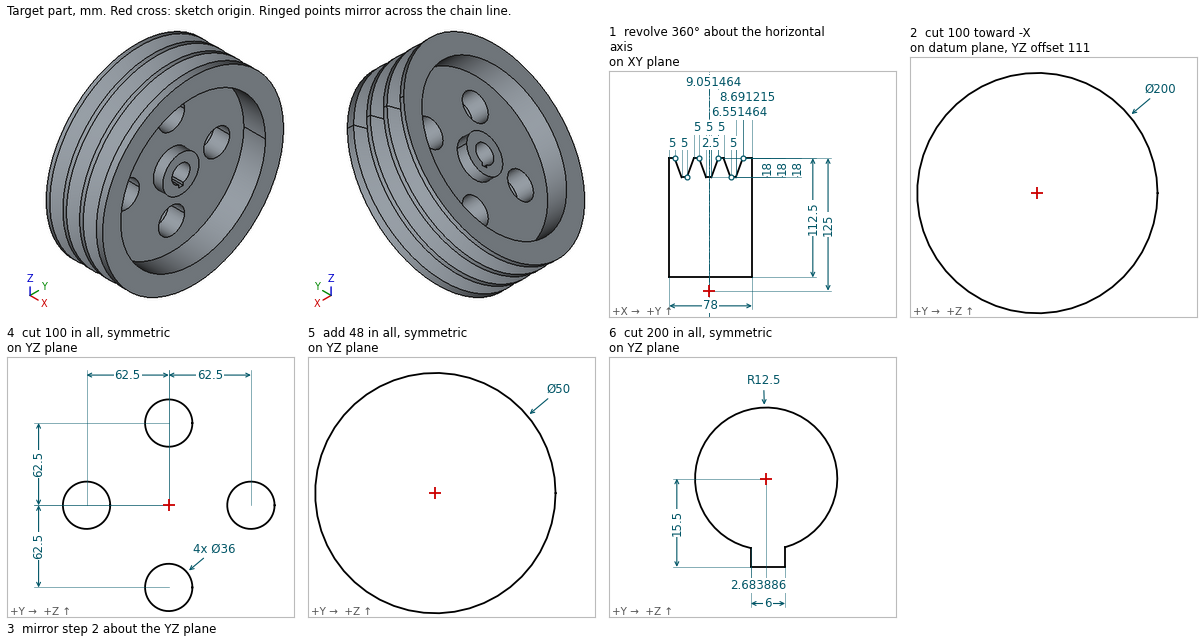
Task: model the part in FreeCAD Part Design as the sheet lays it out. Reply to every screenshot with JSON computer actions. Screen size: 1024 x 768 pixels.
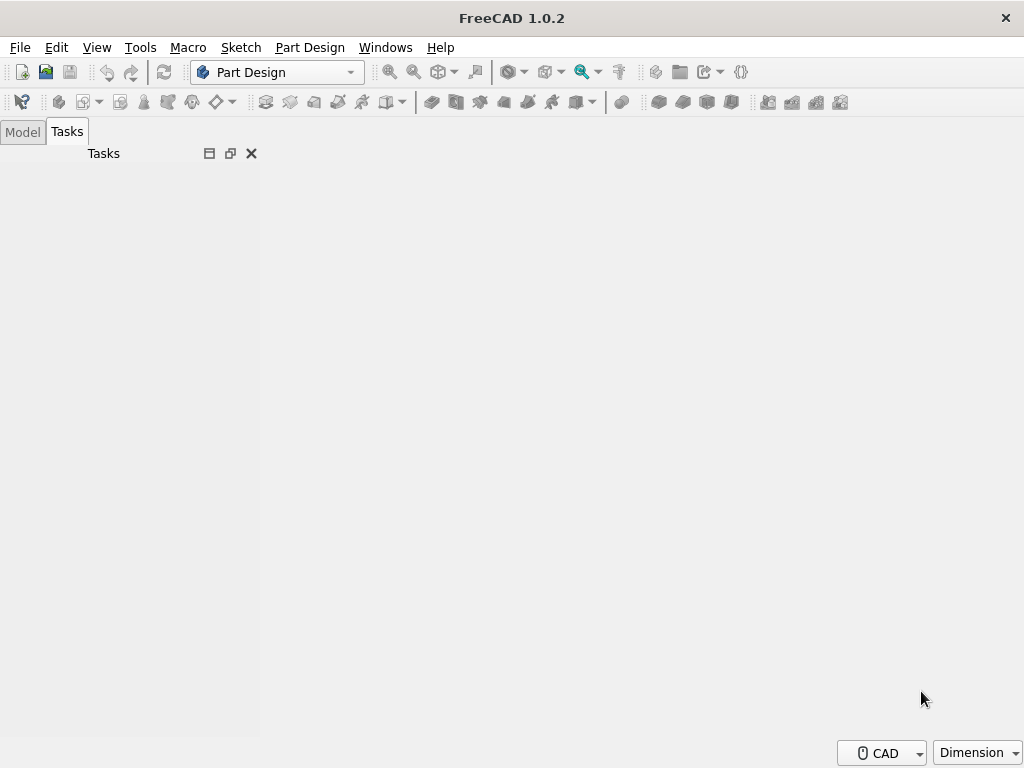
{"action": "left_click", "coordinate": [22, 72]}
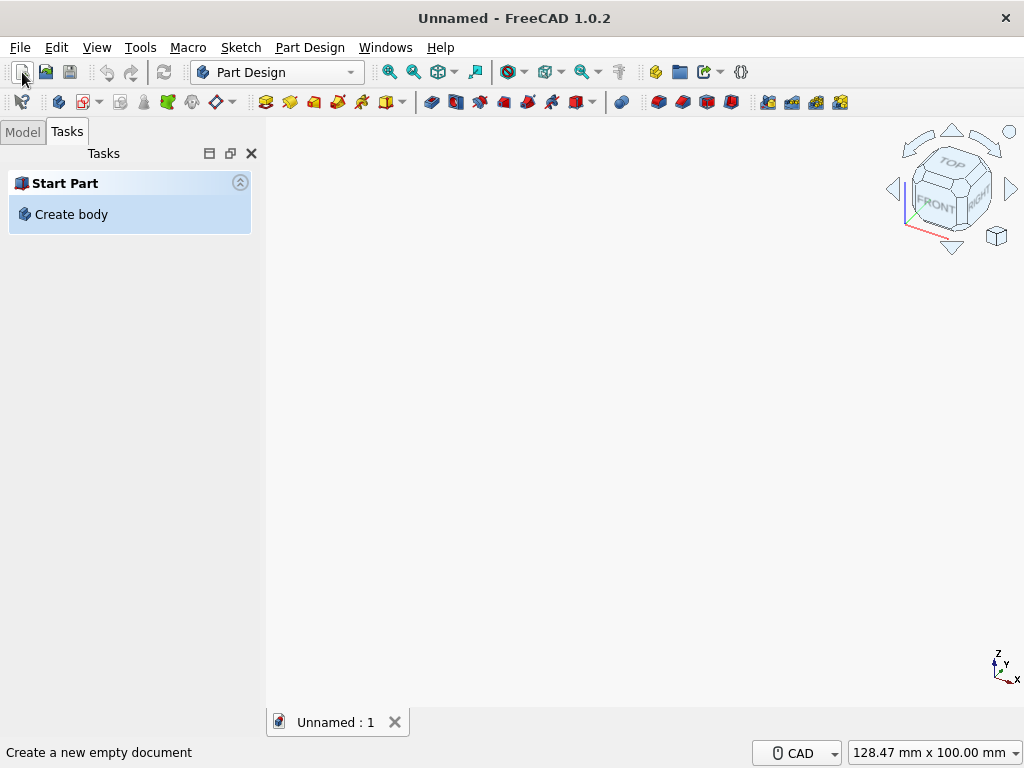
{"action": "left_click", "coordinate": [84, 102]}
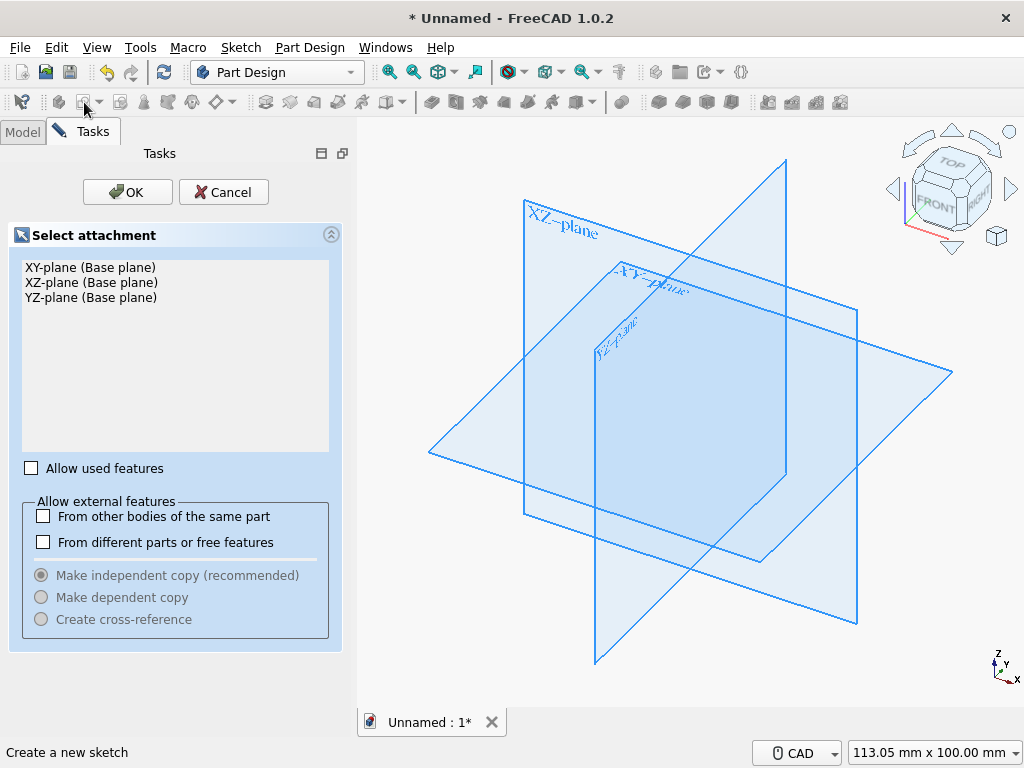
{"action": "left_click", "coordinate": [82, 268]}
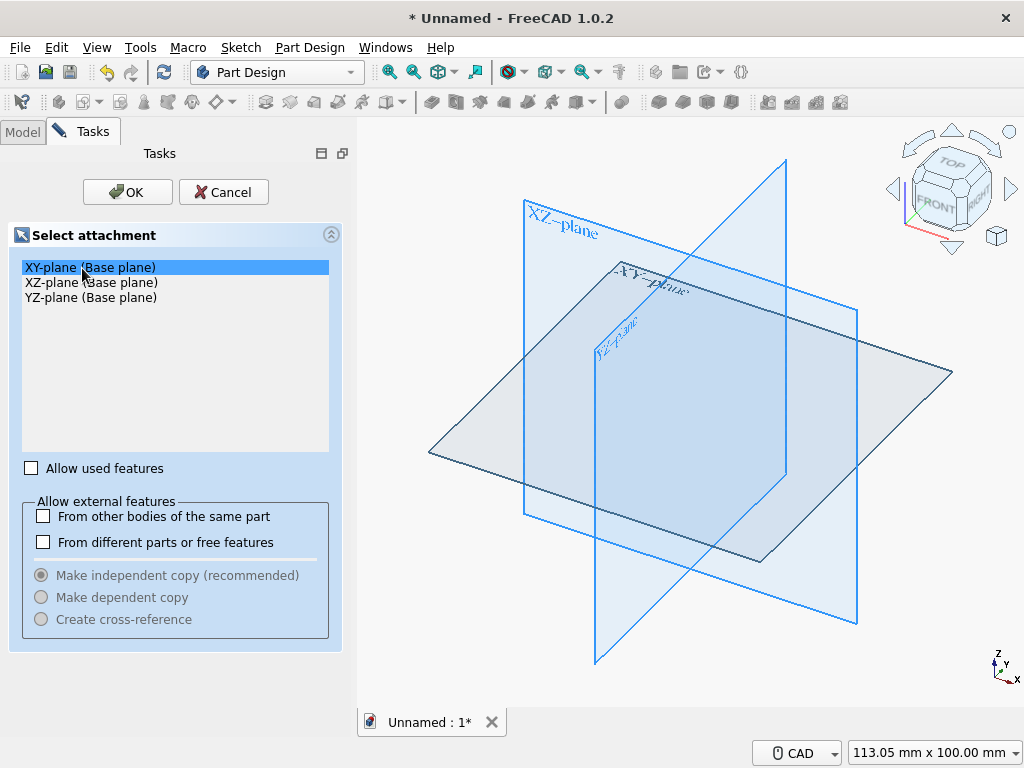
{"action": "left_click", "coordinate": [128, 192]}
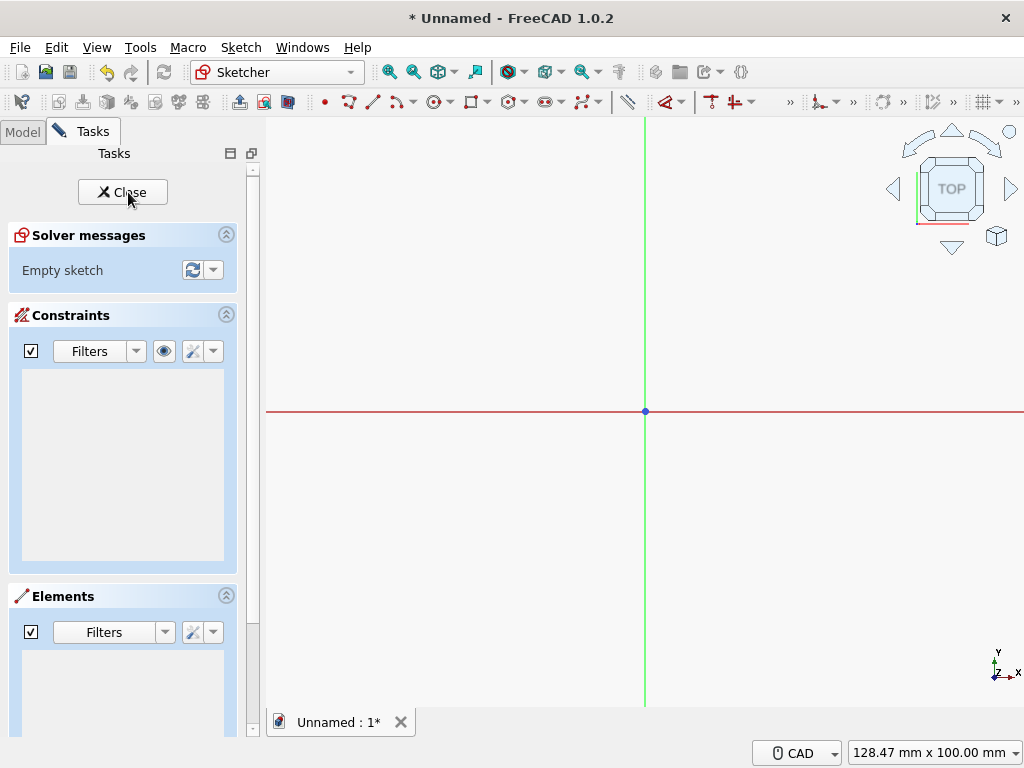
{"action": "scroll", "coordinate": [512, 679], "scroll_direction": "down", "scroll_amount": 4}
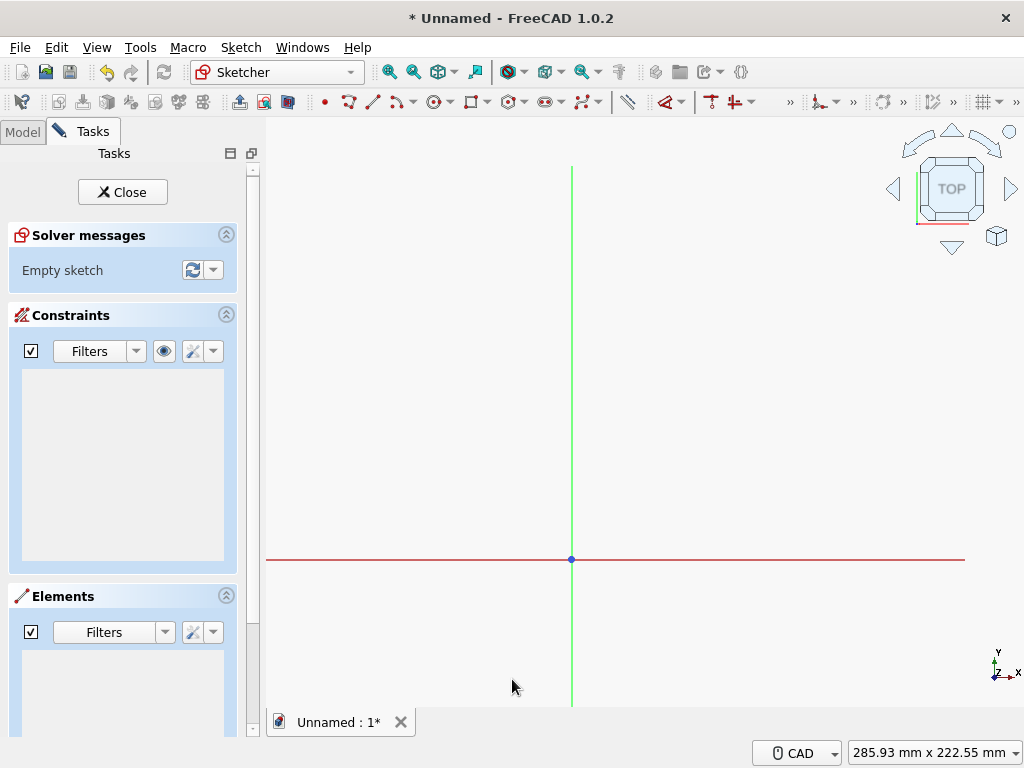
{"action": "left_click", "coordinate": [350, 102]}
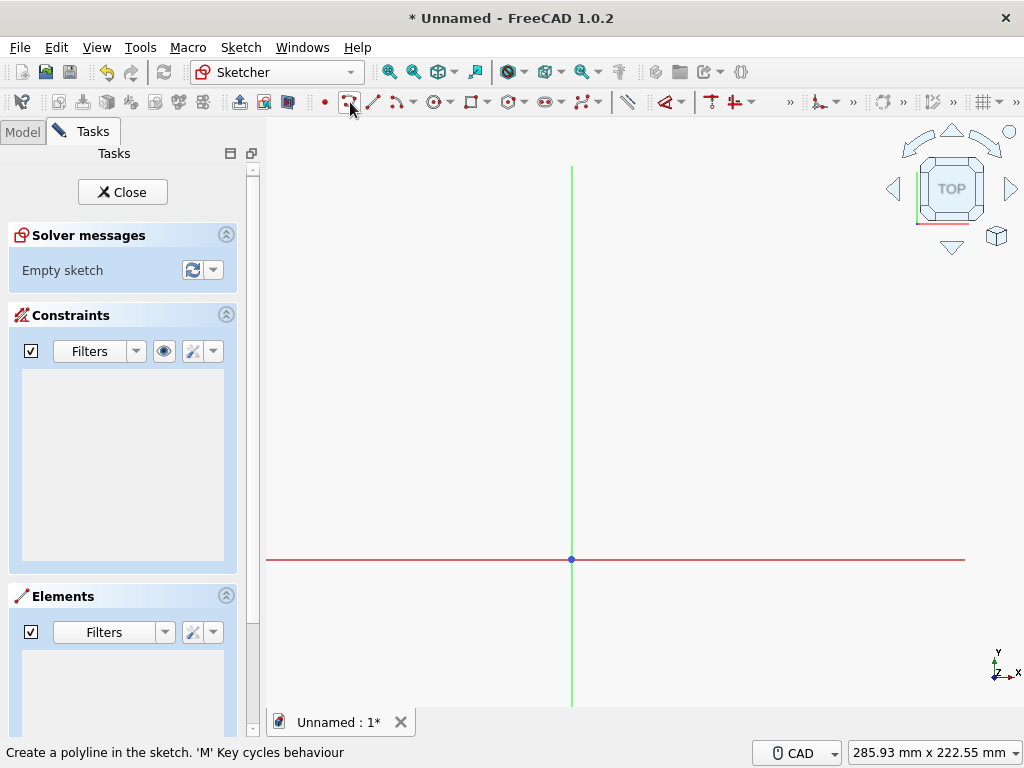
{"action": "left_click", "coordinate": [473, 526]}
{"action": "left_click", "coordinate": [680, 526]}
{"action": "left_click", "coordinate": [680, 228]}
{"action": "left_click", "coordinate": [657, 228]}
{"action": "left_click", "coordinate": [640, 276]}
{"action": "left_click", "coordinate": [627, 276]}
{"action": "left_click", "coordinate": [609, 228]}
{"action": "left_click", "coordinate": [596, 228]}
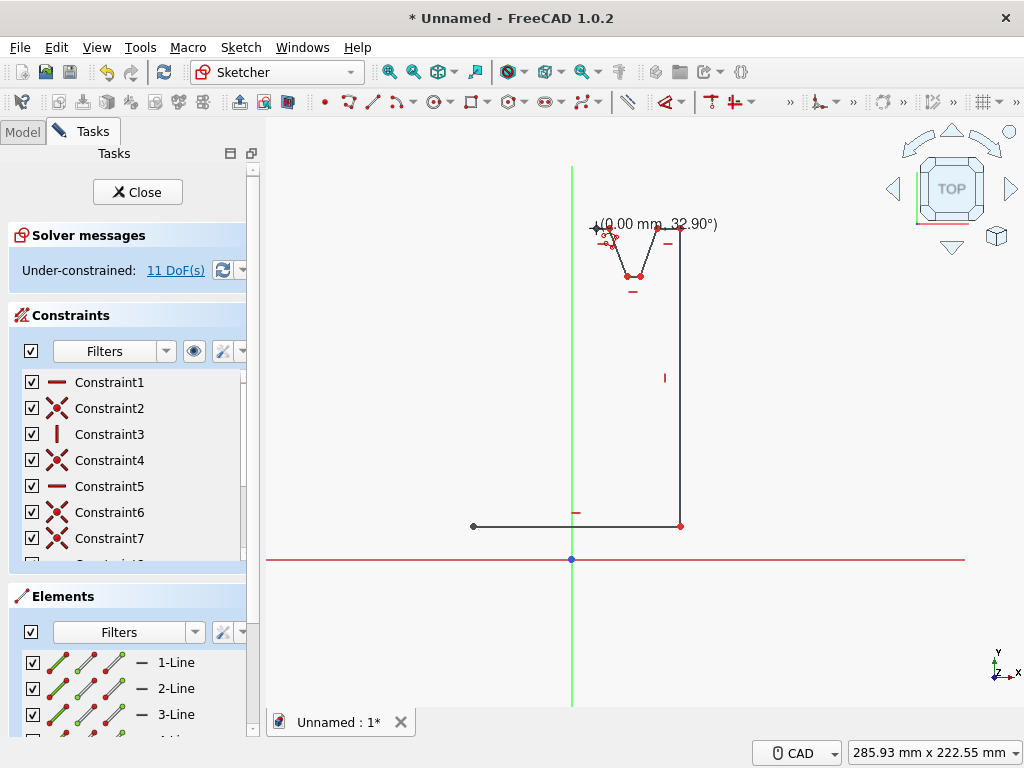
{"action": "scroll", "coordinate": [579, 276], "scroll_direction": "up", "scroll_amount": 5}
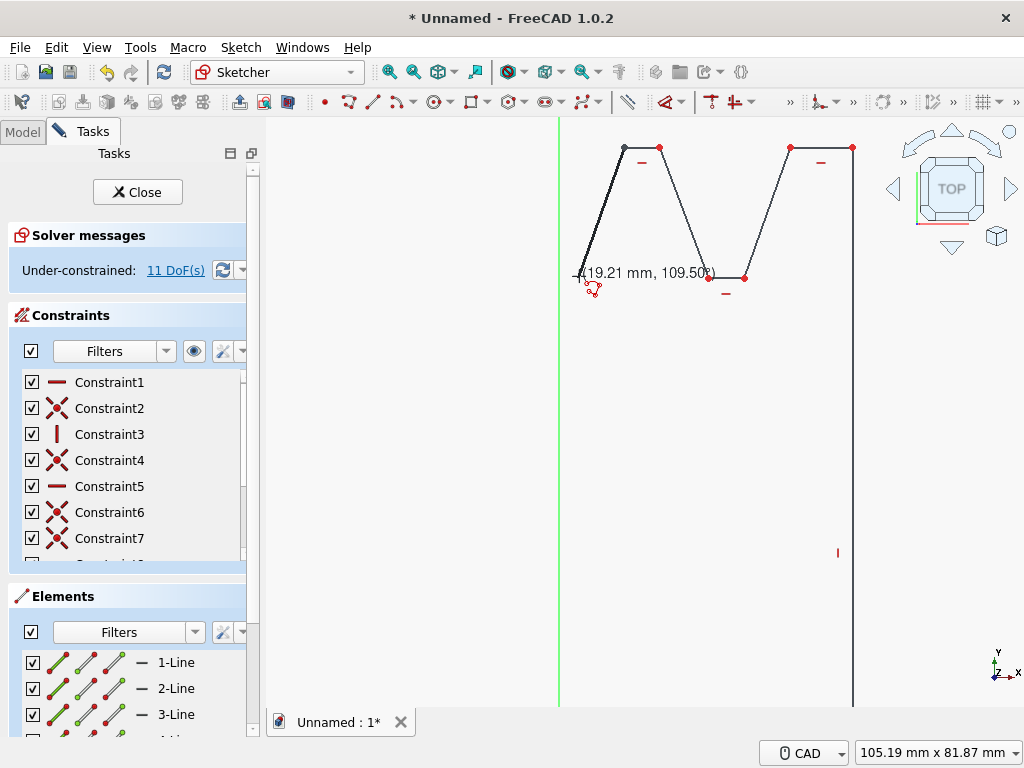
{"action": "left_click", "coordinate": [577, 275]}
{"action": "left_click", "coordinate": [541, 275]}
{"action": "left_click", "coordinate": [494, 146]}
{"action": "left_click", "coordinate": [458, 146]}
{"action": "left_click", "coordinate": [411, 275]}
{"action": "left_click", "coordinate": [375, 275]}
{"action": "left_click", "coordinate": [327, 146]}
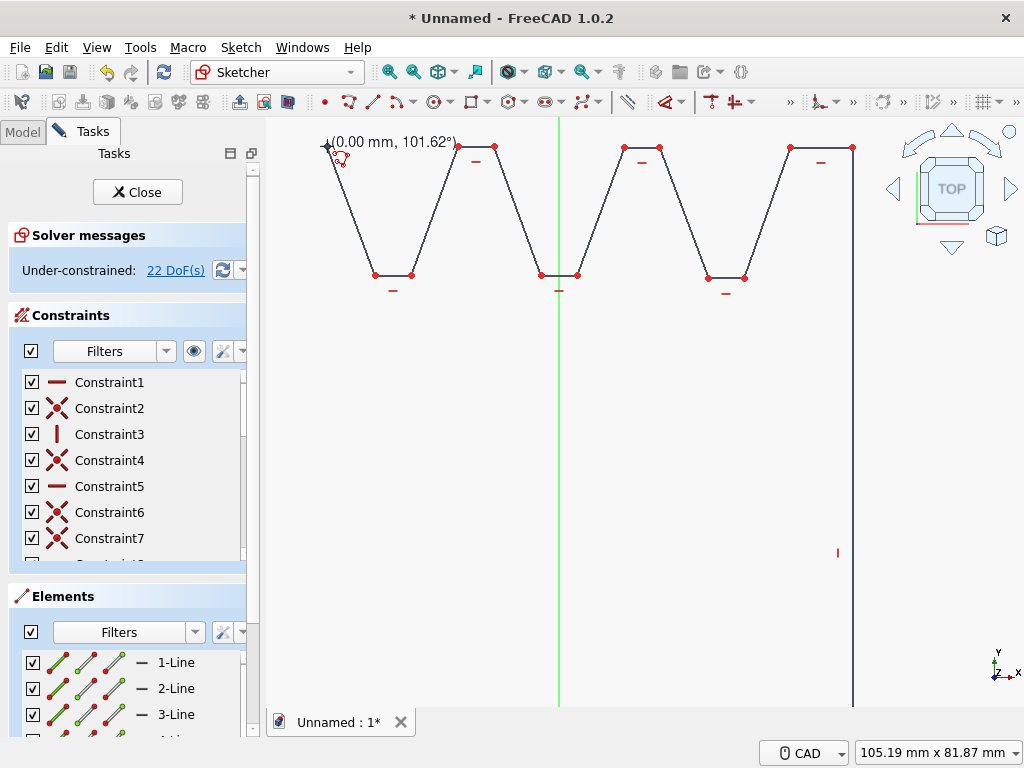
{"action": "scroll", "coordinate": [580, 262], "scroll_direction": "down", "scroll_amount": 4}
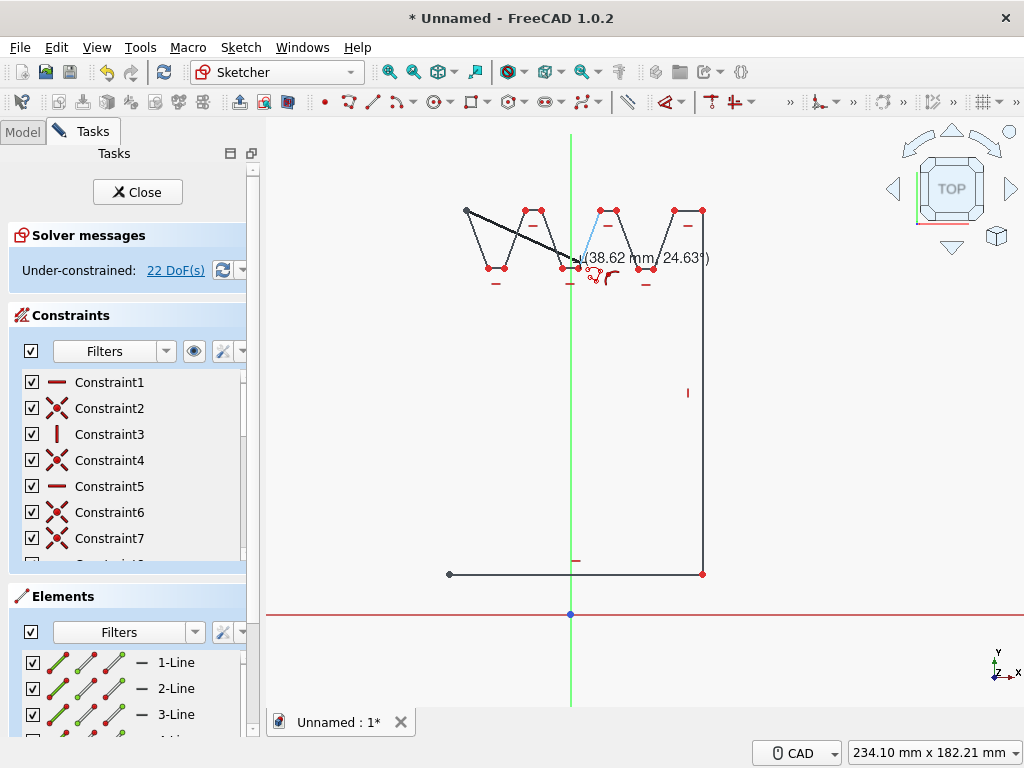
{"action": "left_click", "coordinate": [451, 210]}
{"action": "left_click", "coordinate": [450, 575]}
{"action": "key", "text": "Escape"}
{"action": "key", "text": "Escape"}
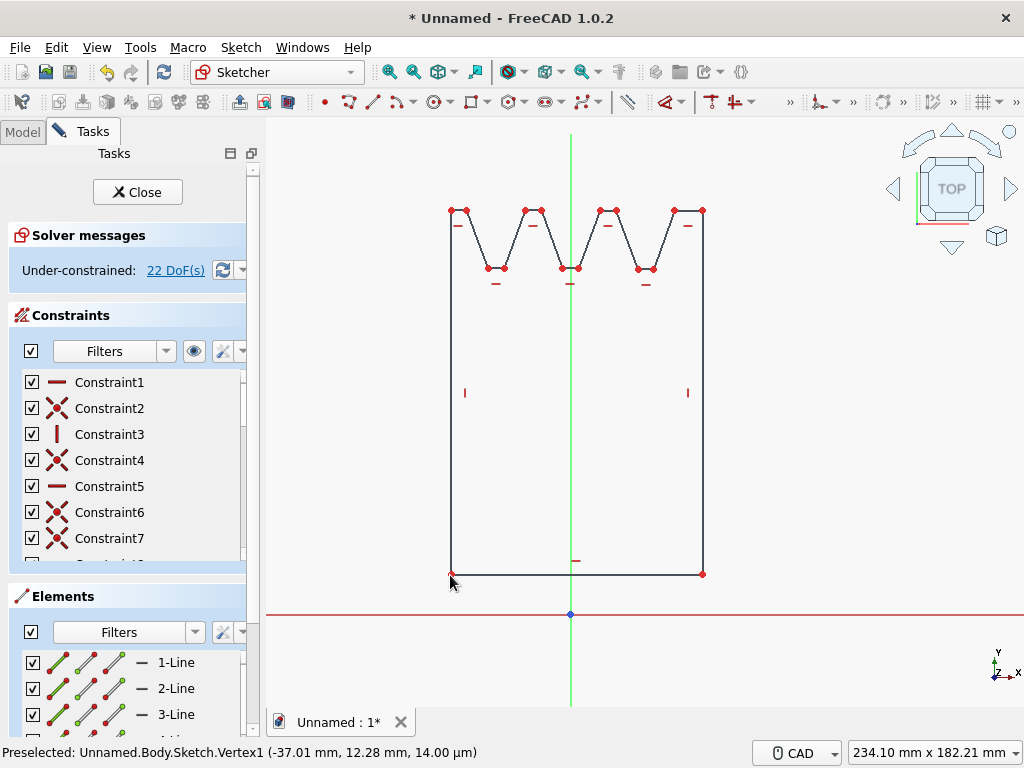
{"action": "left_click", "coordinate": [600, 211]}